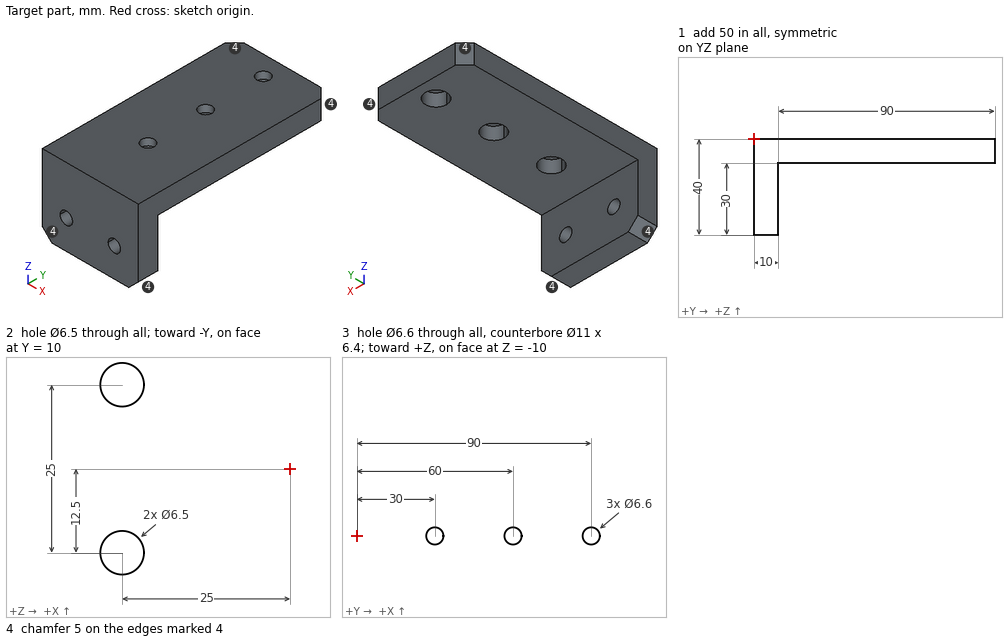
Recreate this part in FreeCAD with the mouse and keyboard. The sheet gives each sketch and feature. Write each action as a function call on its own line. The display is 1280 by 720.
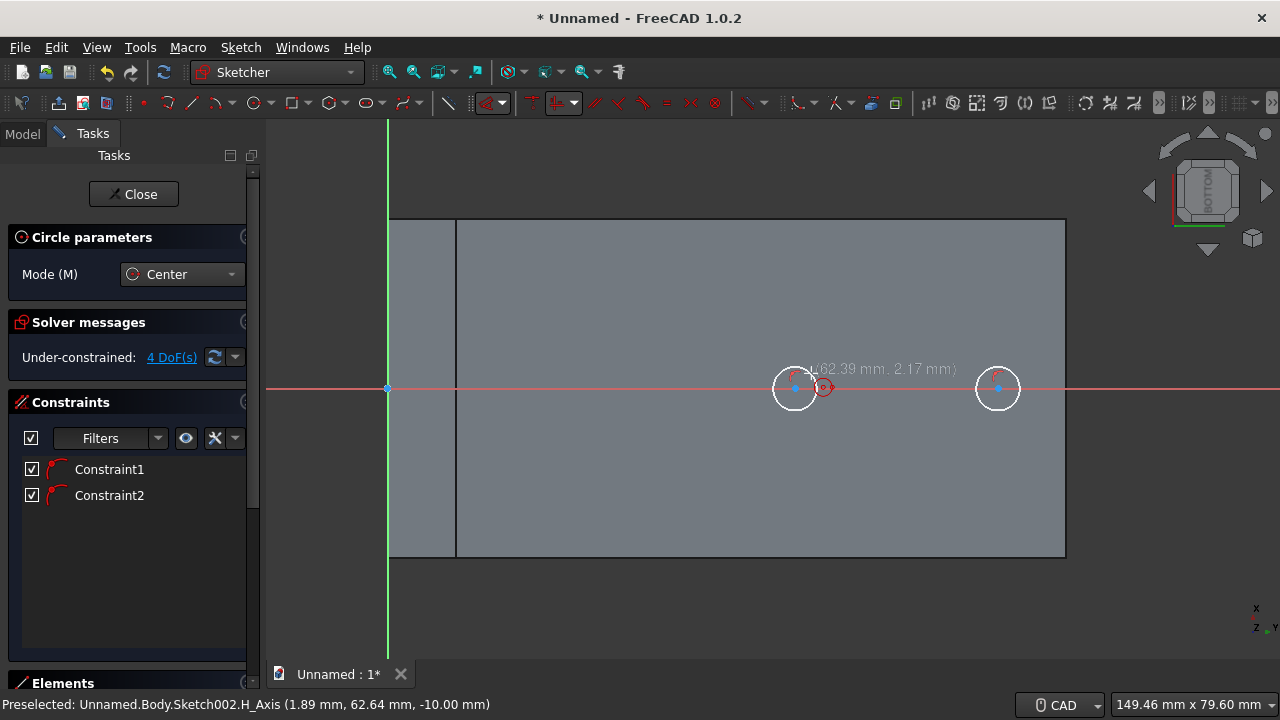
click(591, 389)
click(607, 373)
key(Escape)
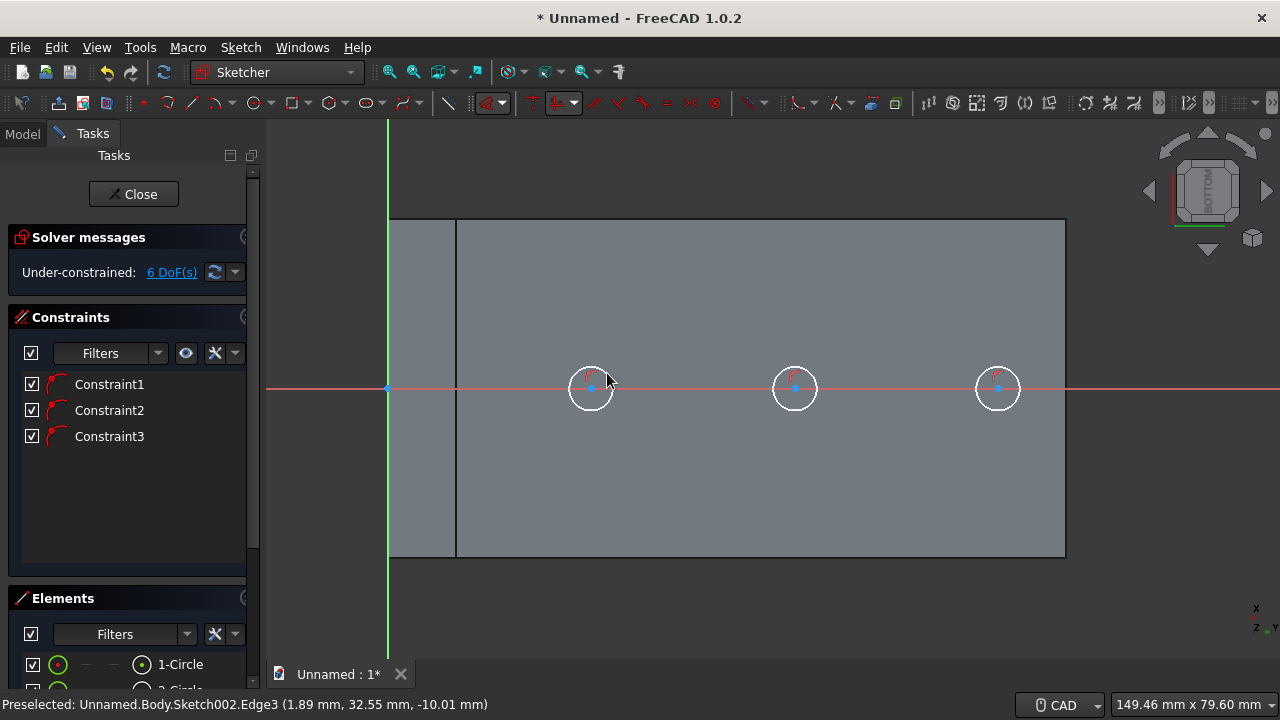
click(1013, 373)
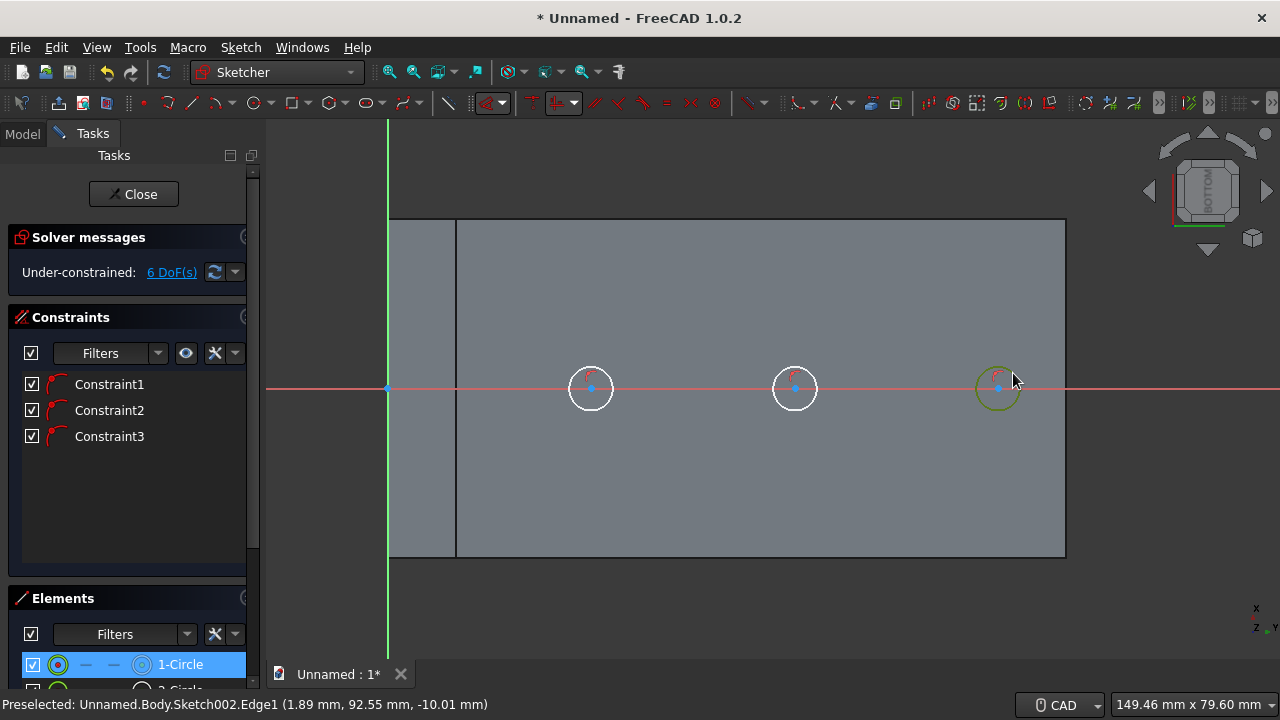
click(810, 373)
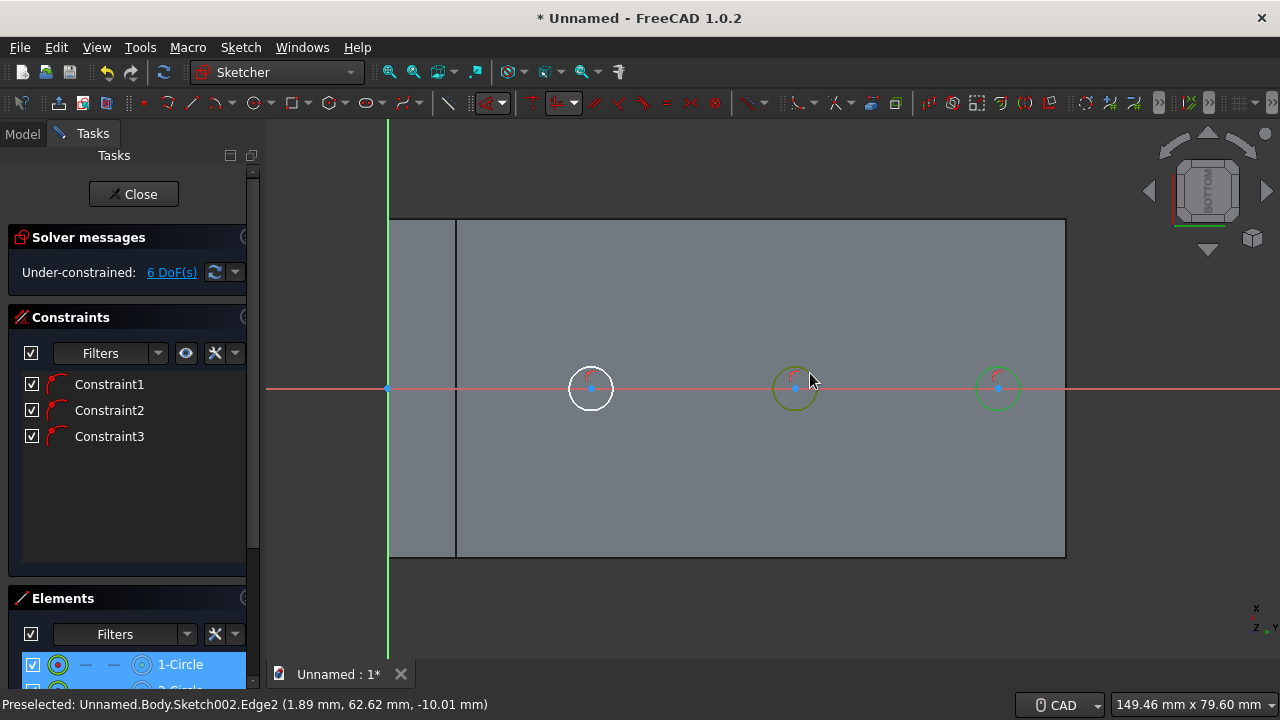
click(606, 373)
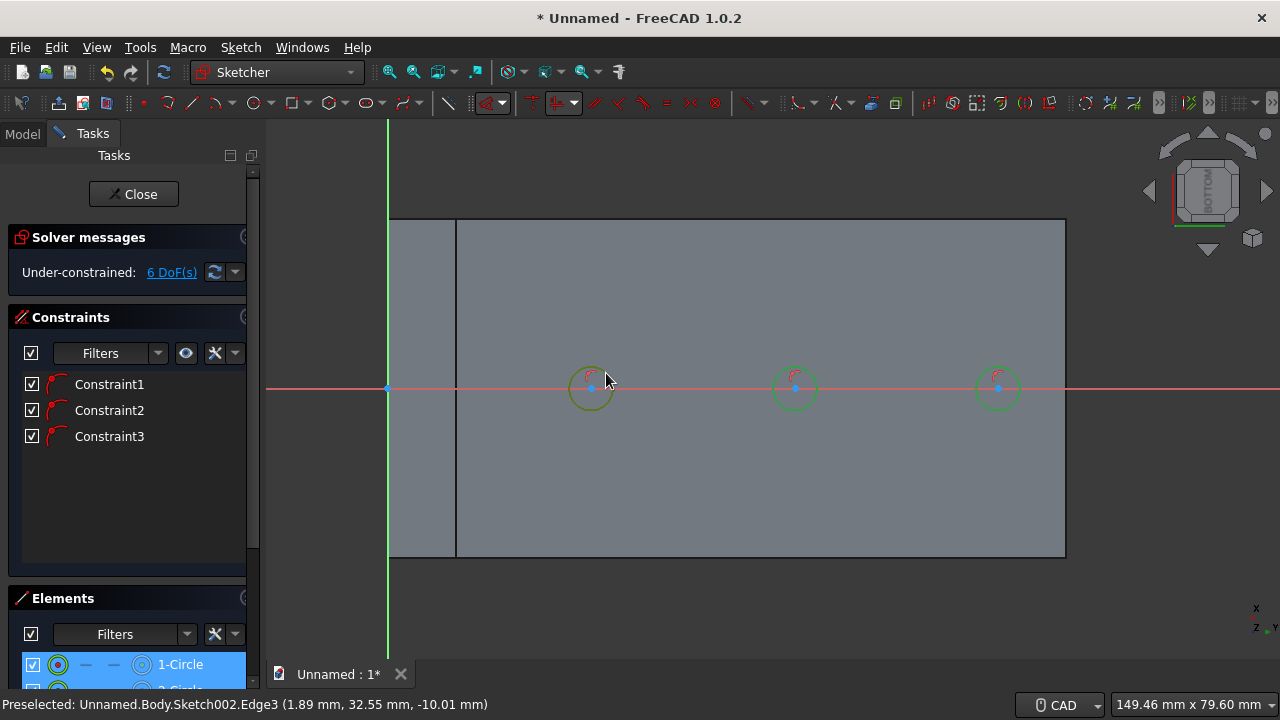
click(668, 104)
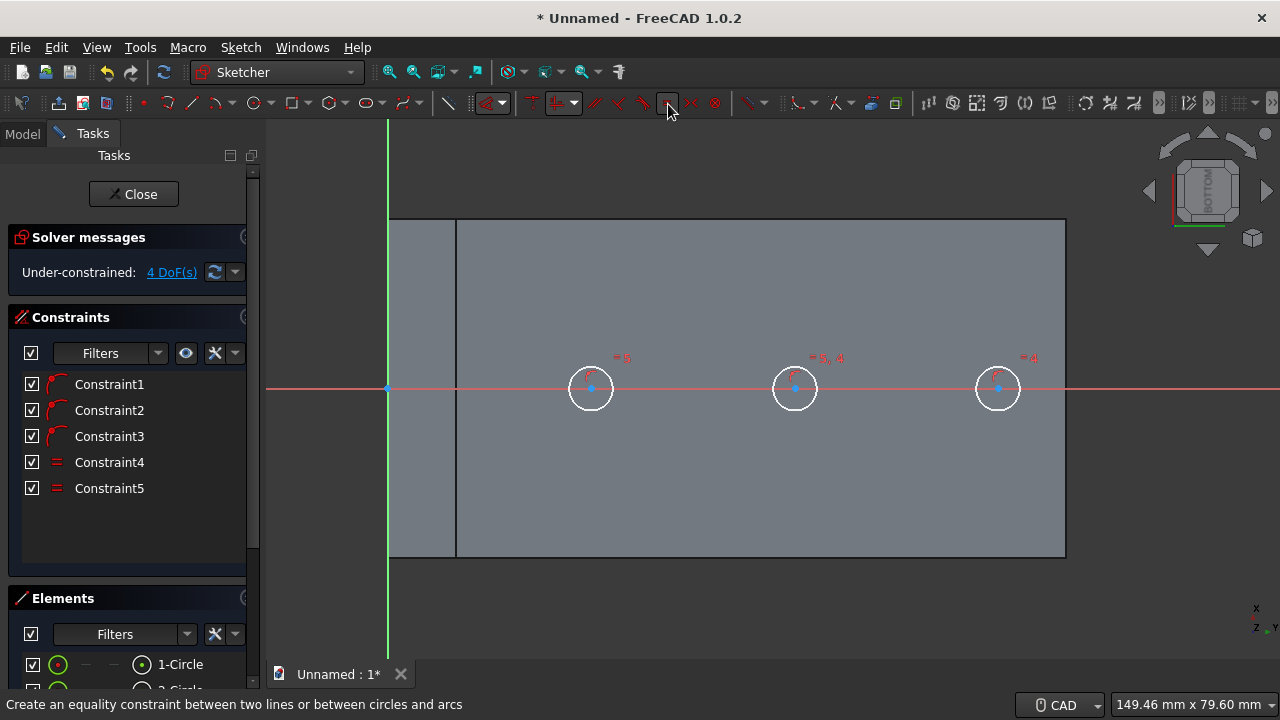
click(1013, 373)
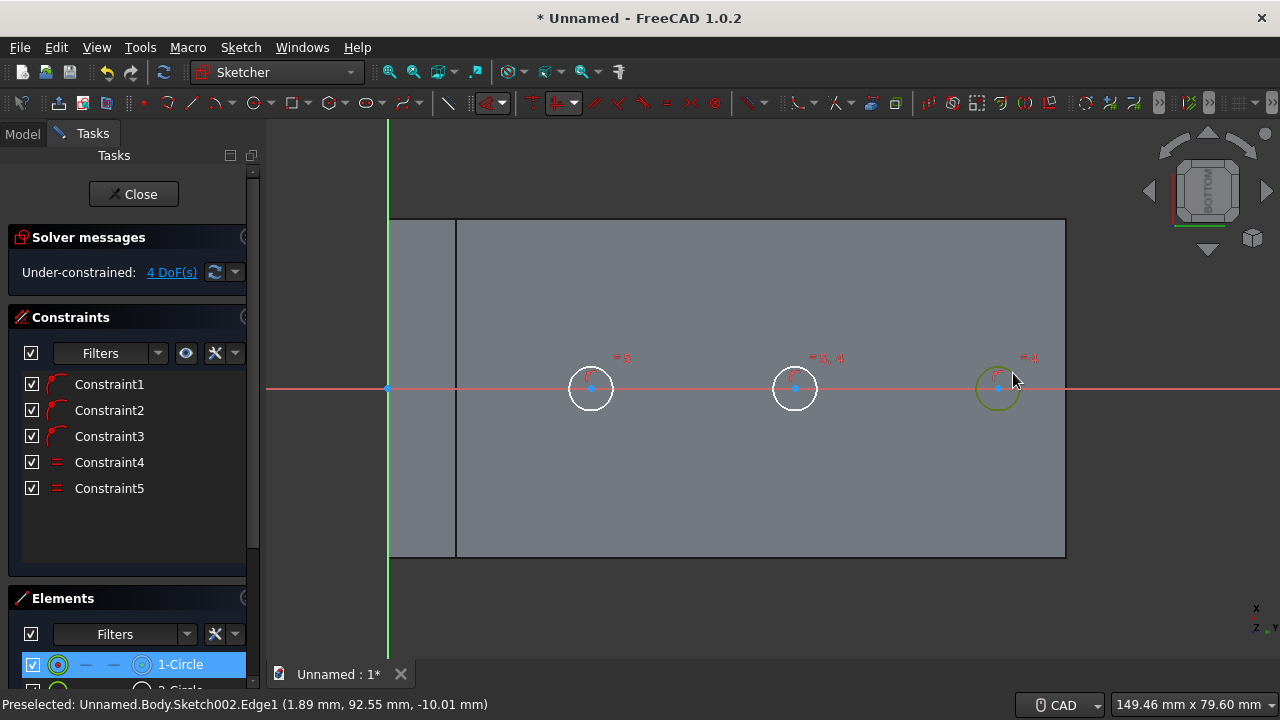
click(504, 104)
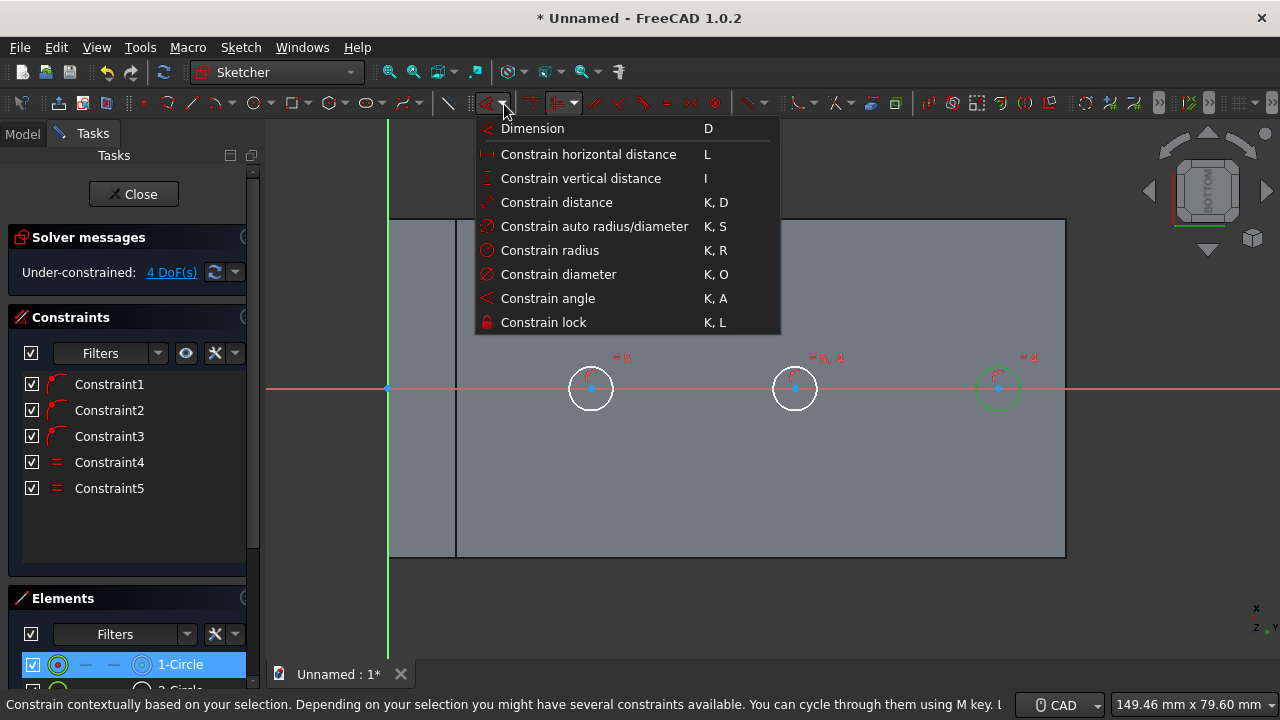
click(628, 274)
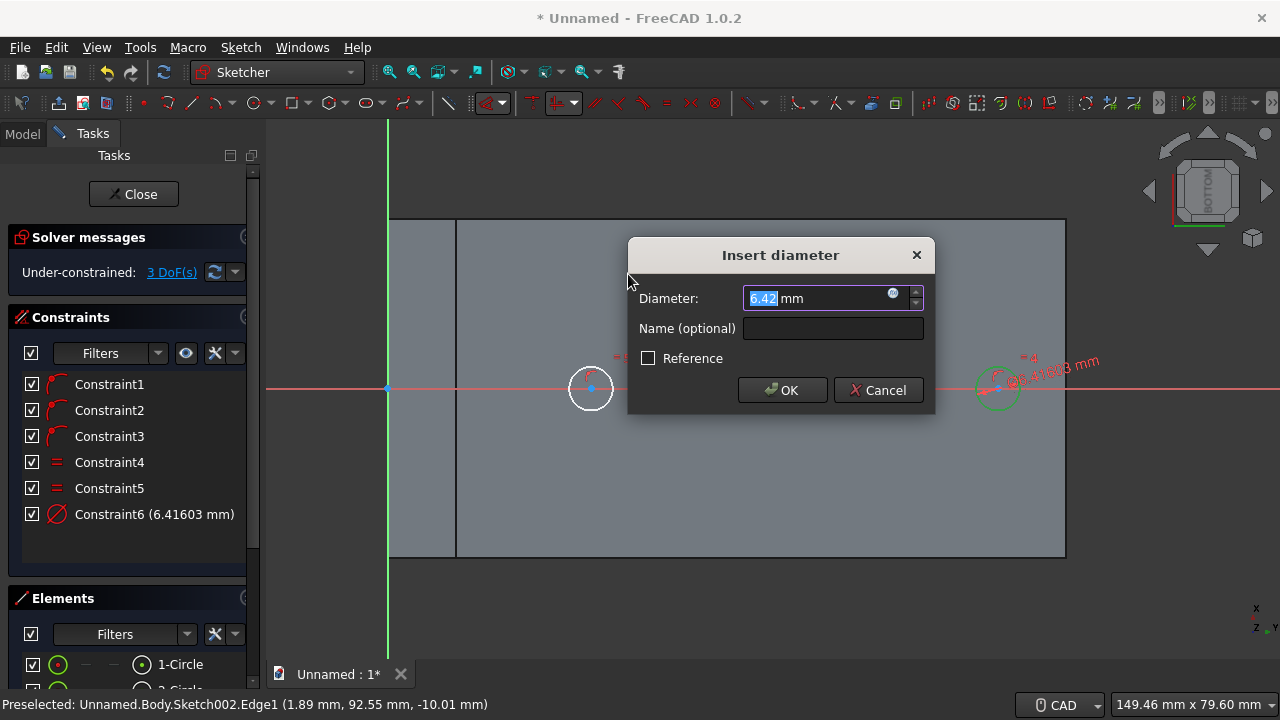
text(6.6)
key(Return)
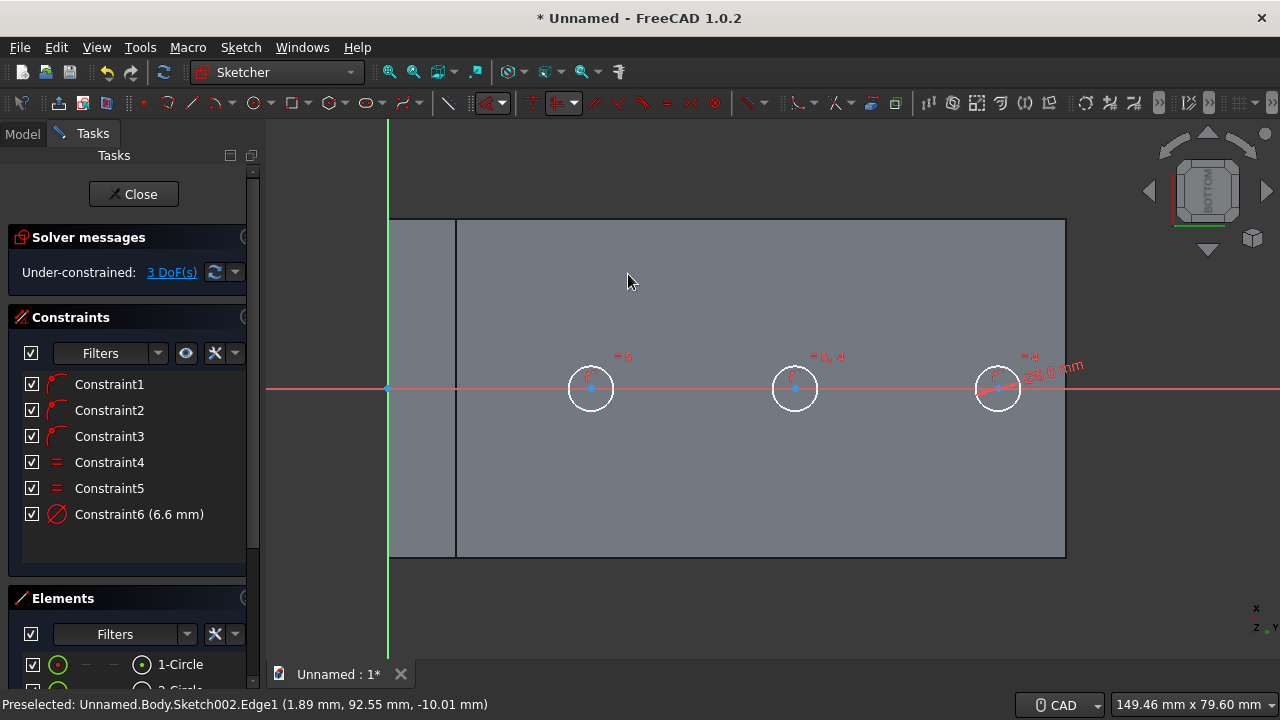
click(998, 389)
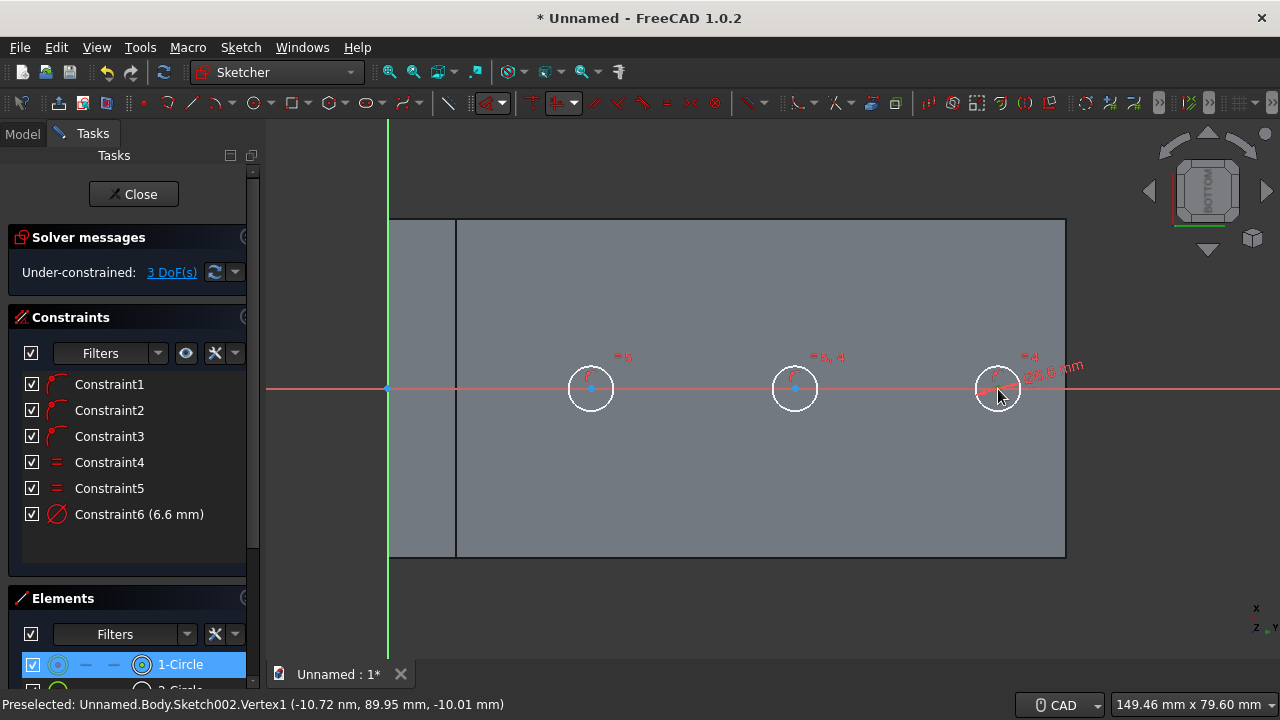
click(504, 104)